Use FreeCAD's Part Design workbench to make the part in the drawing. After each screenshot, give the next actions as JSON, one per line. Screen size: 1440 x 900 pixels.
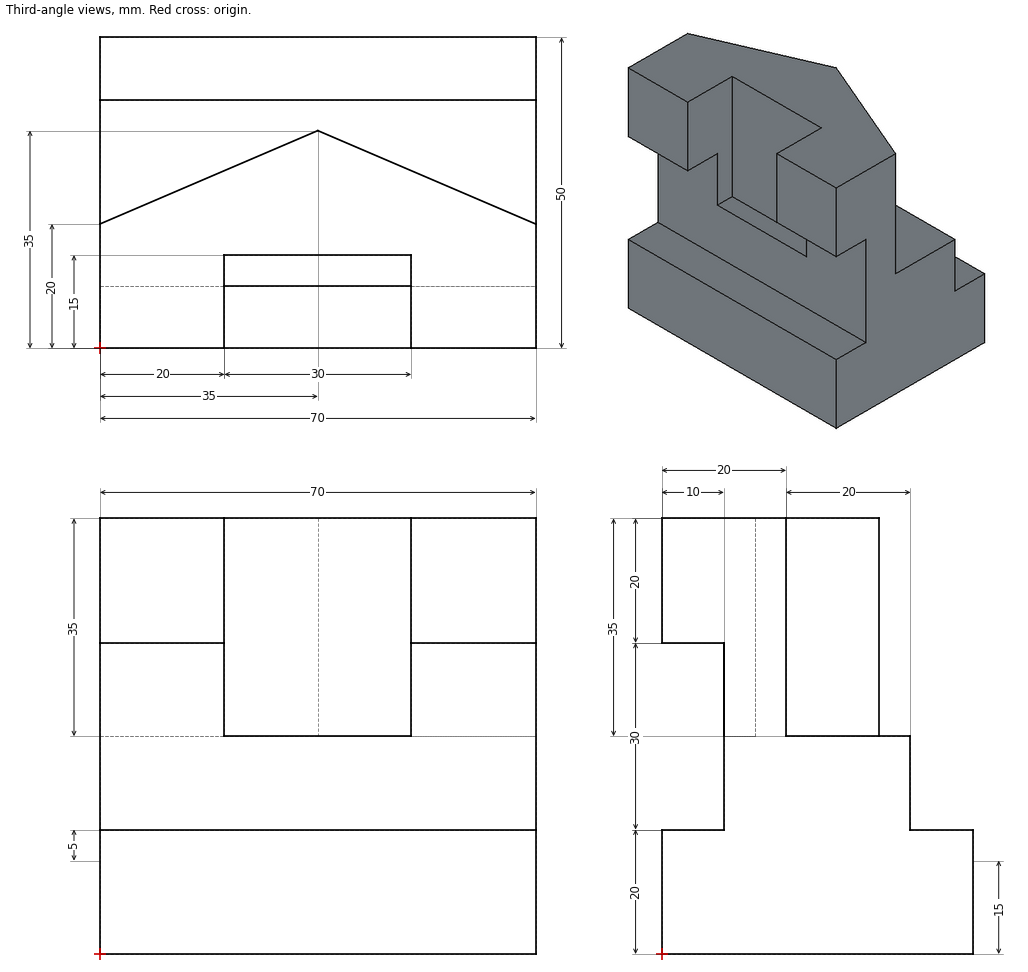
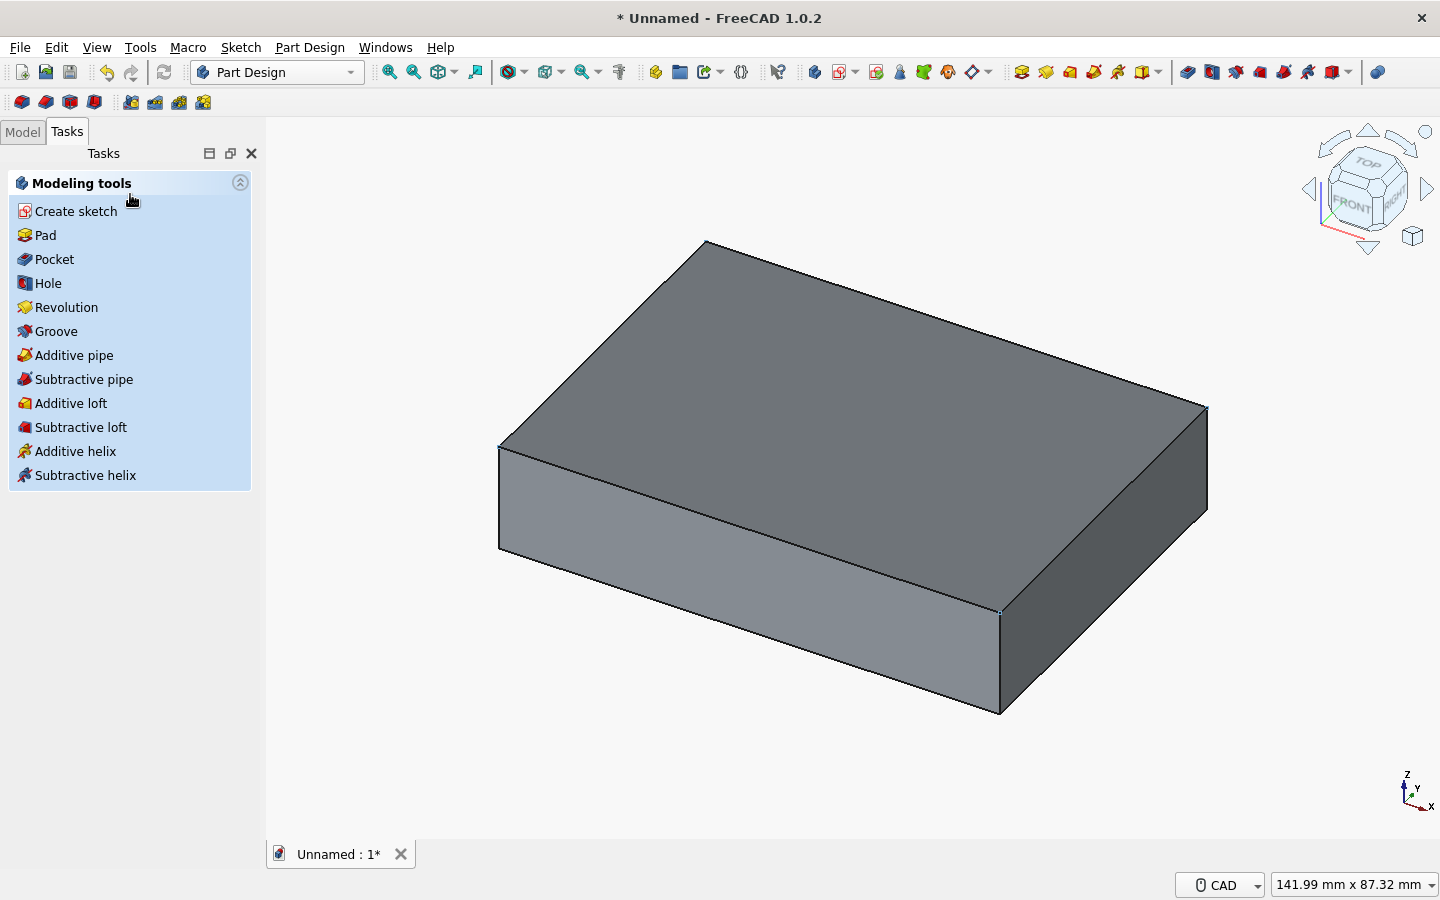
{"action": "left_click", "coordinate": [1022, 72]}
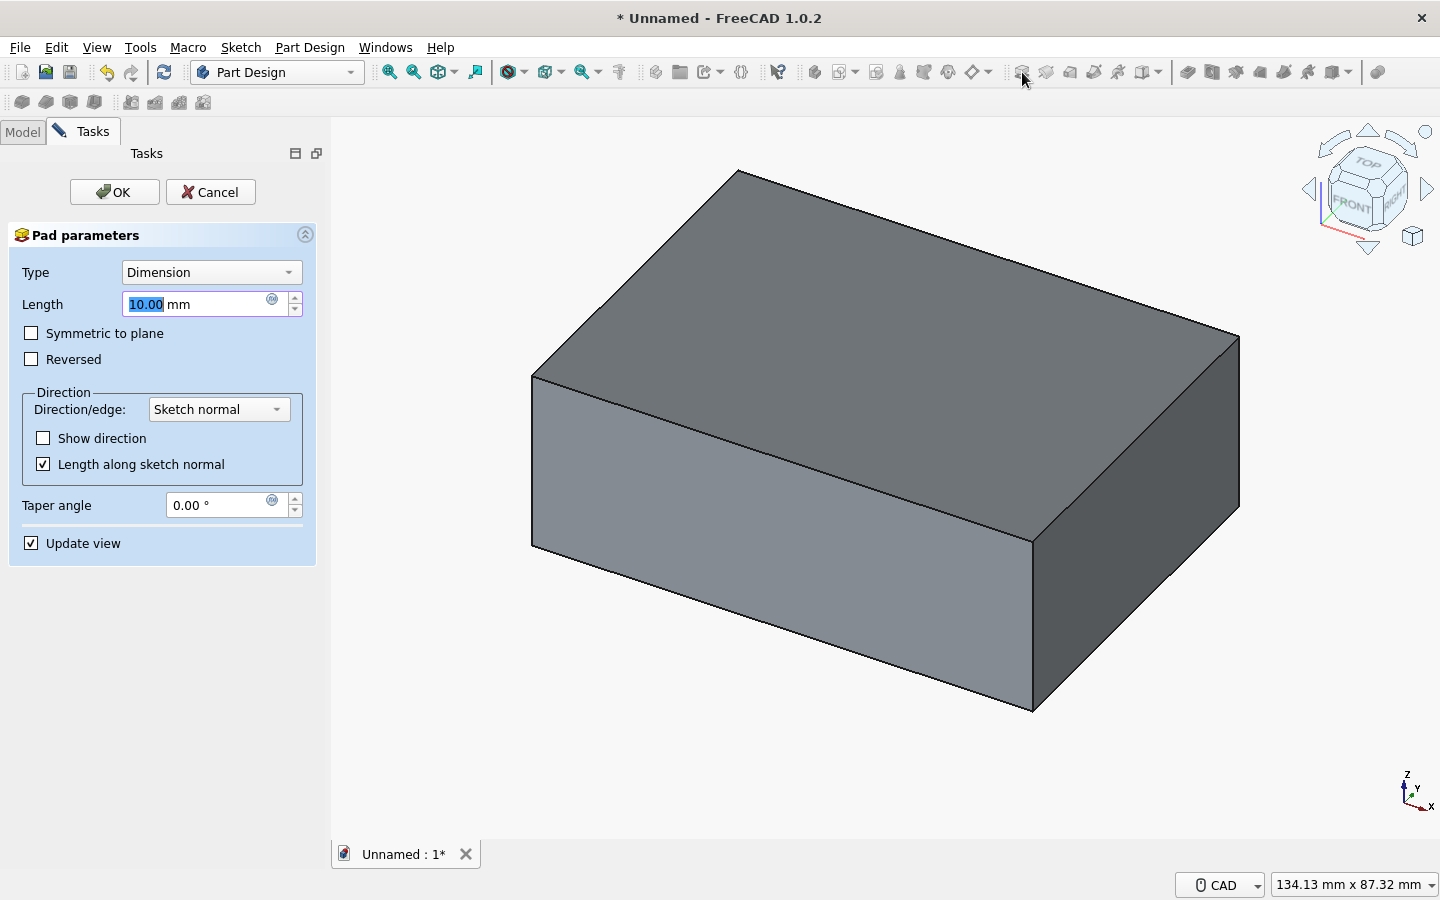
{"action": "type", "text": "5"}
{"action": "key", "text": "Tab"}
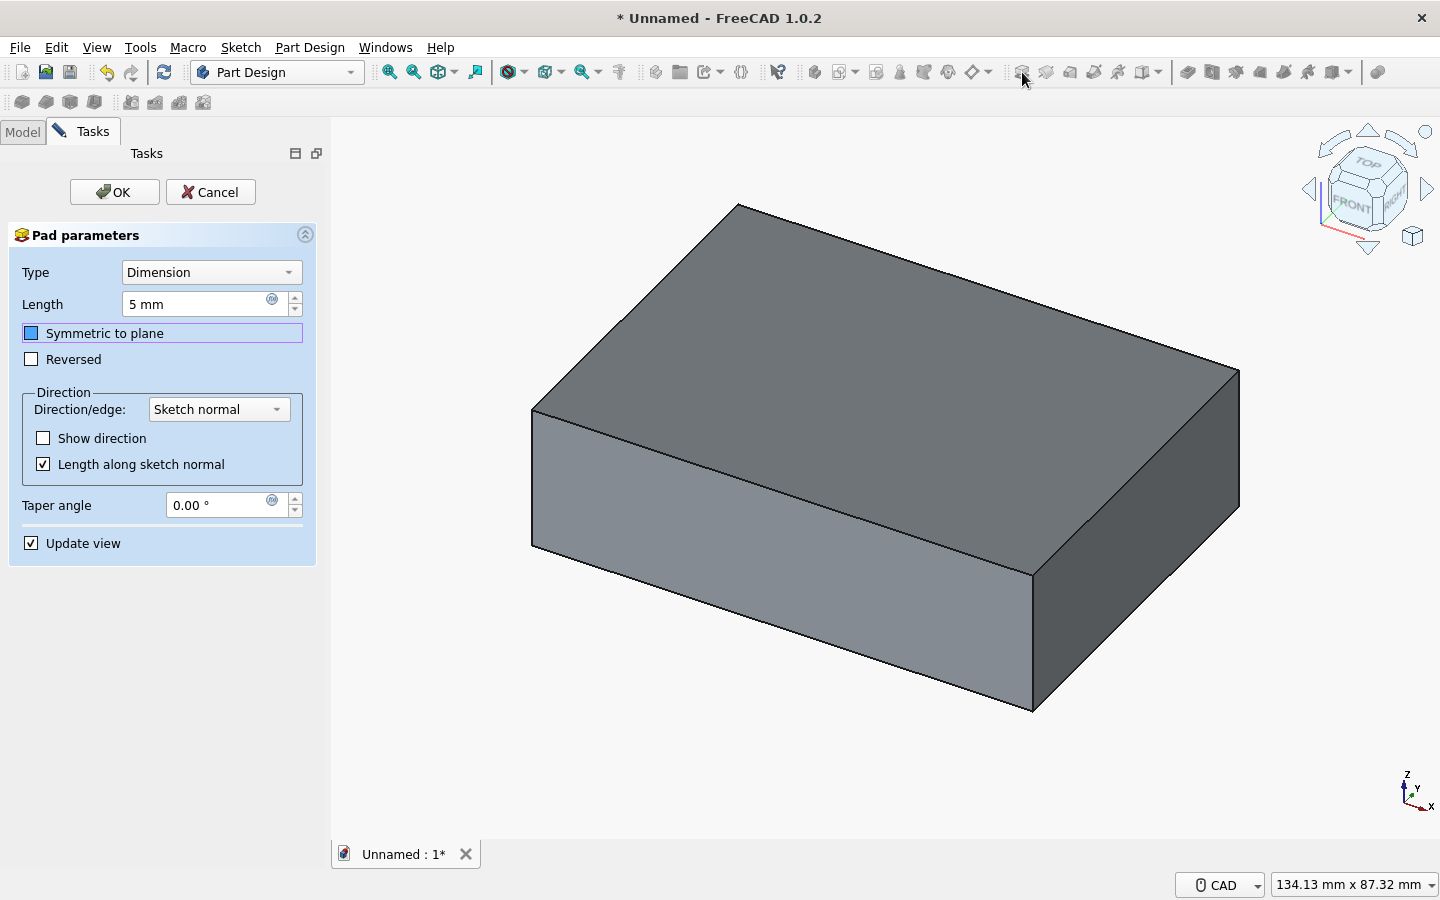
{"action": "left_click", "coordinate": [115, 192]}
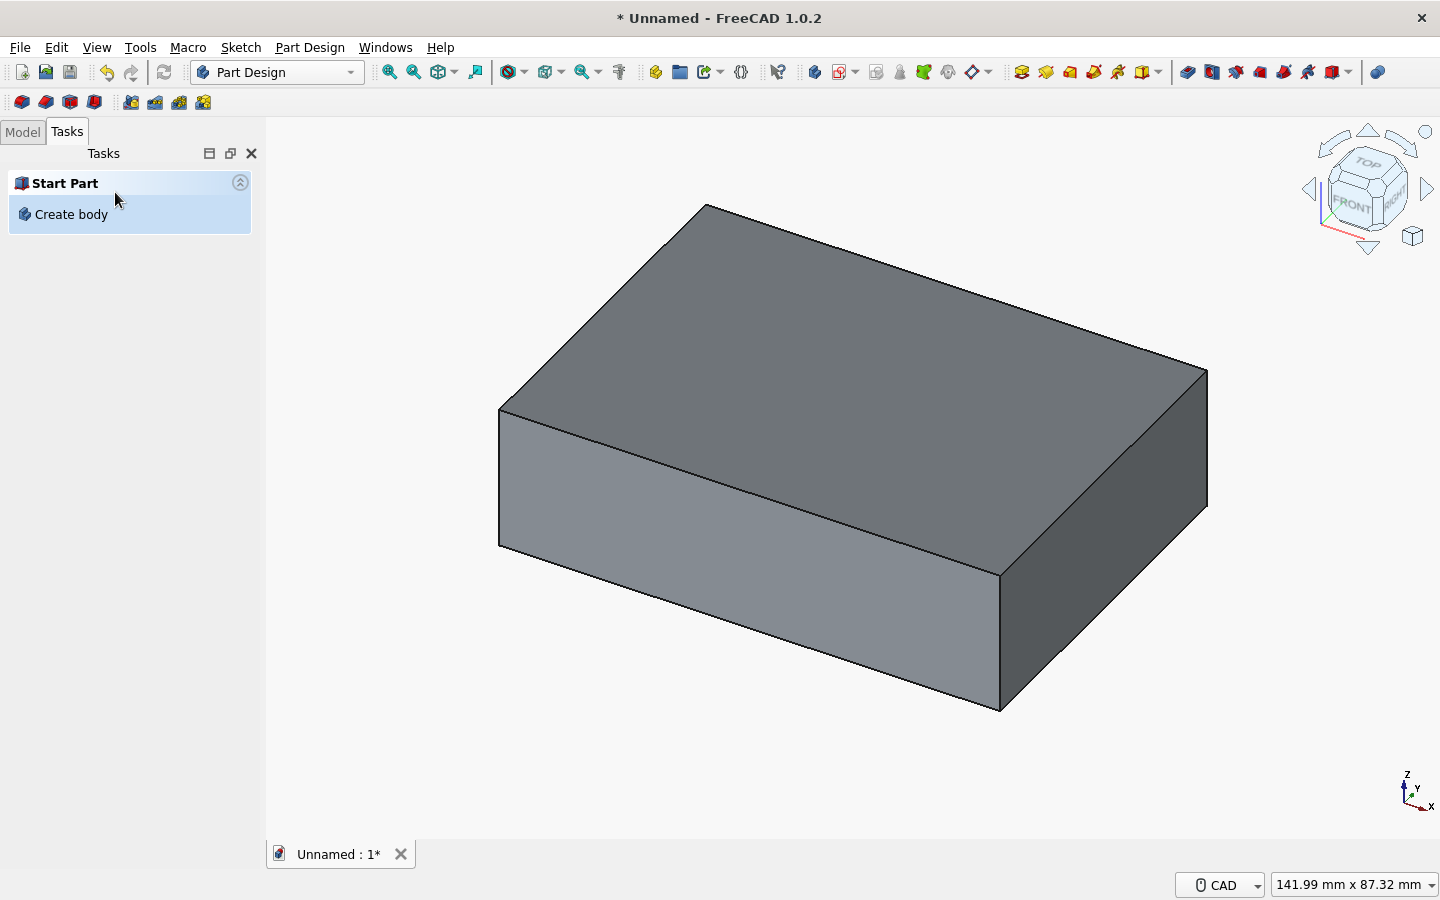
{"action": "key", "text": "6"}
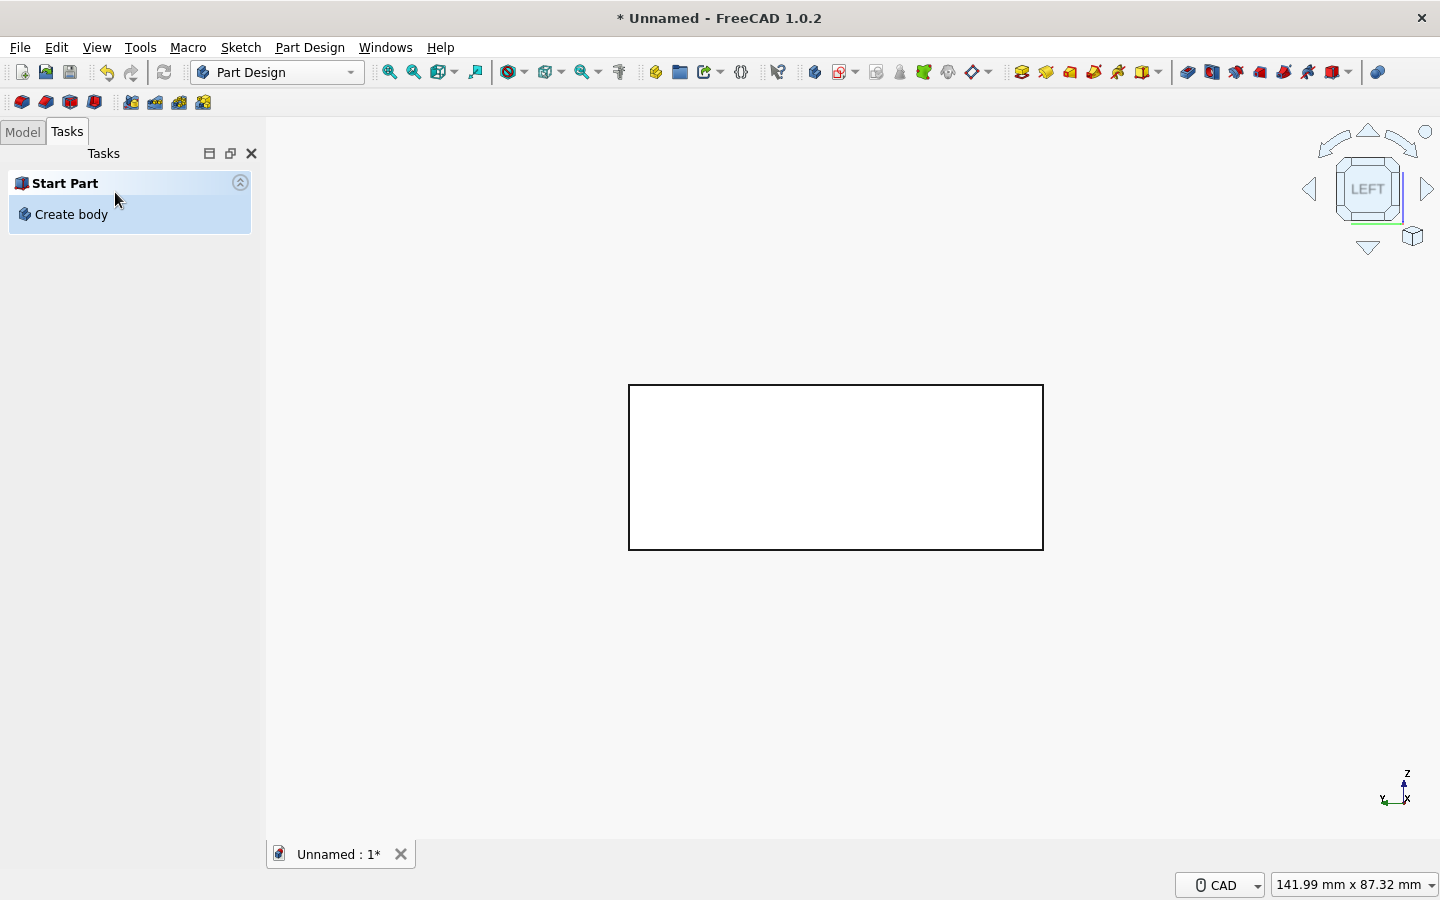
{"action": "left_click", "coordinate": [390, 72]}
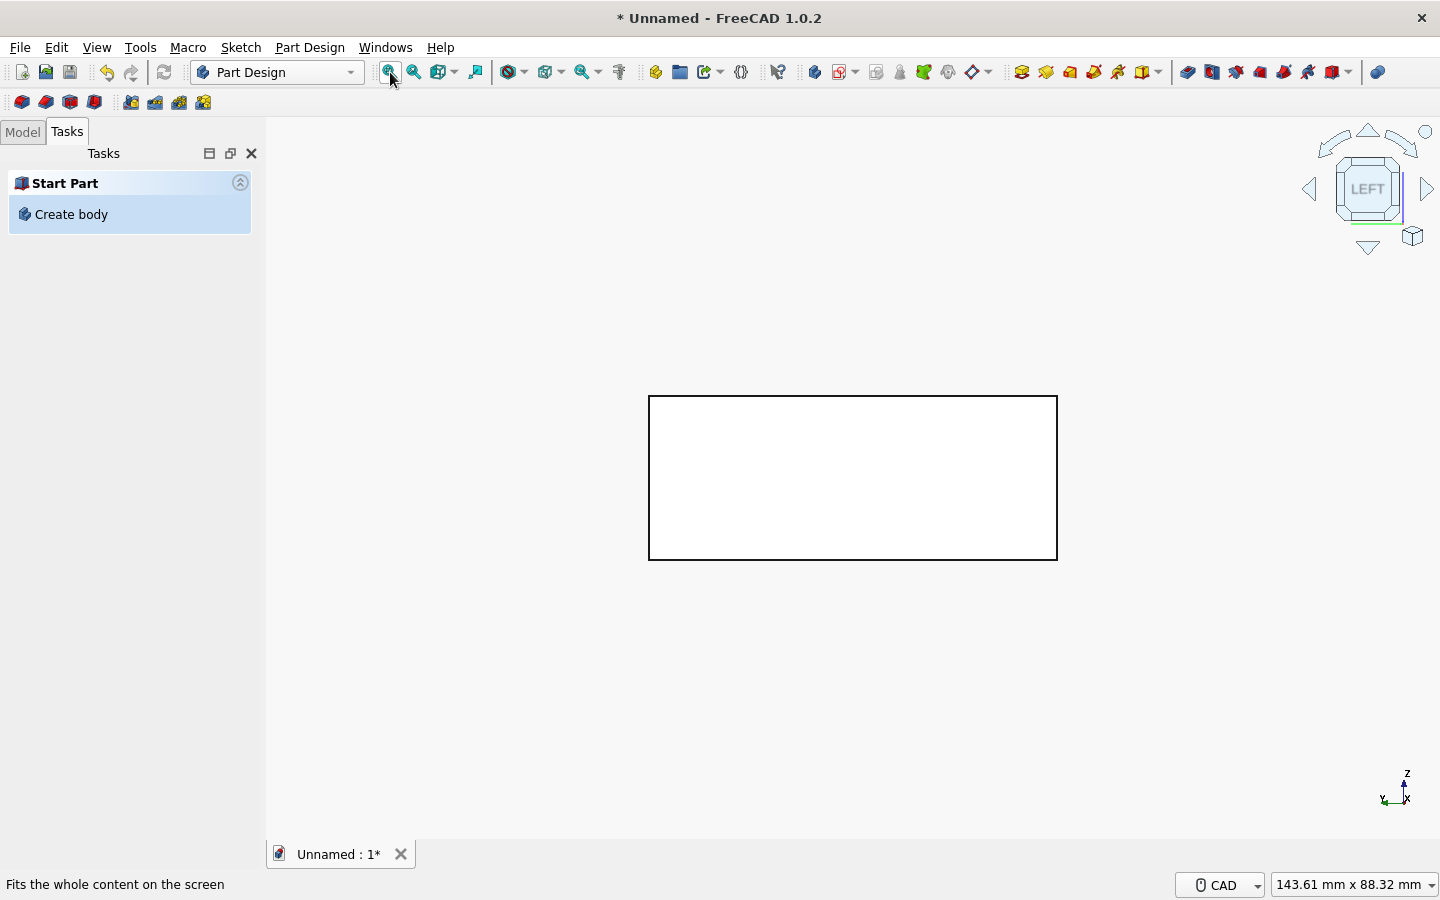
{"action": "left_click", "coordinate": [736, 477]}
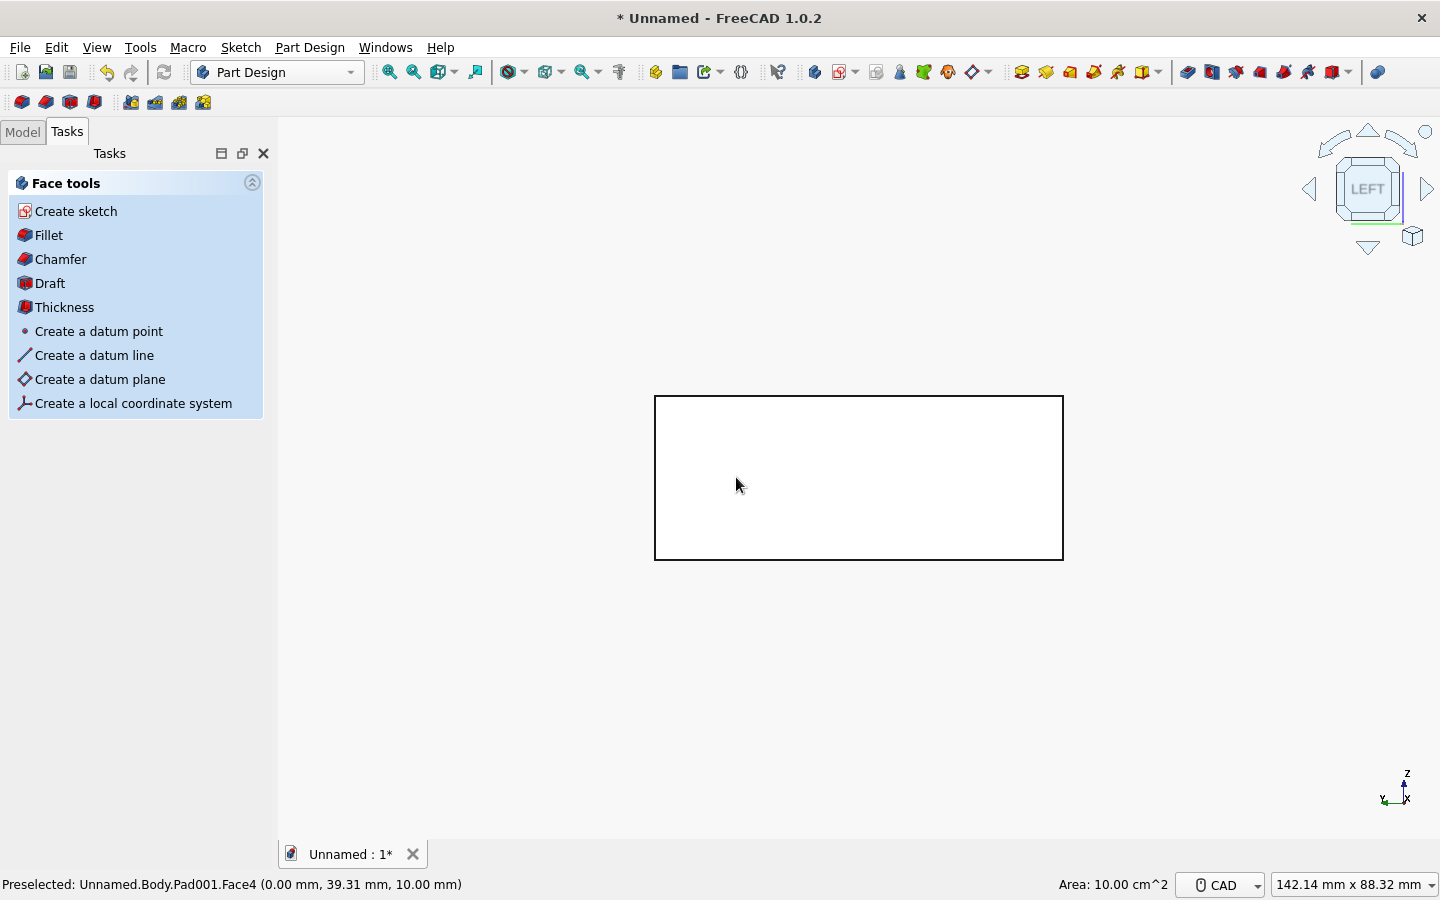
{"action": "left_click", "coordinate": [840, 72]}